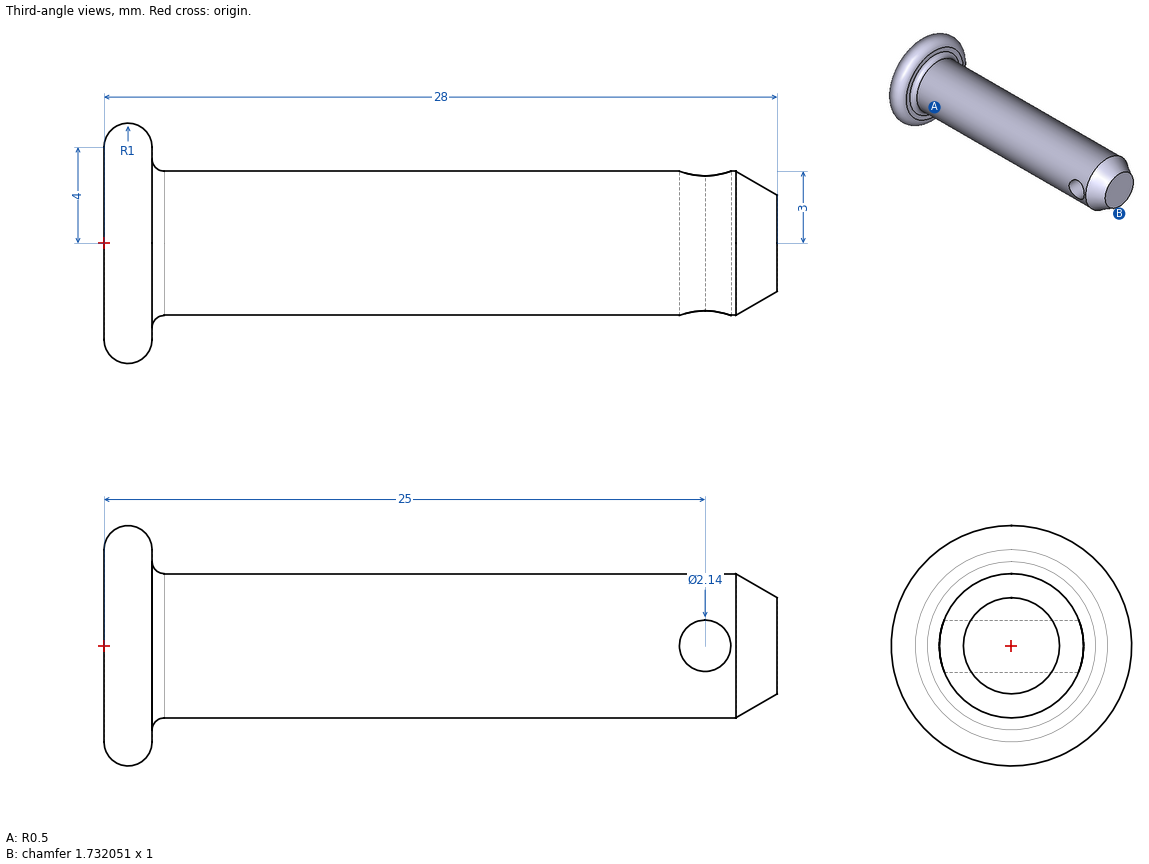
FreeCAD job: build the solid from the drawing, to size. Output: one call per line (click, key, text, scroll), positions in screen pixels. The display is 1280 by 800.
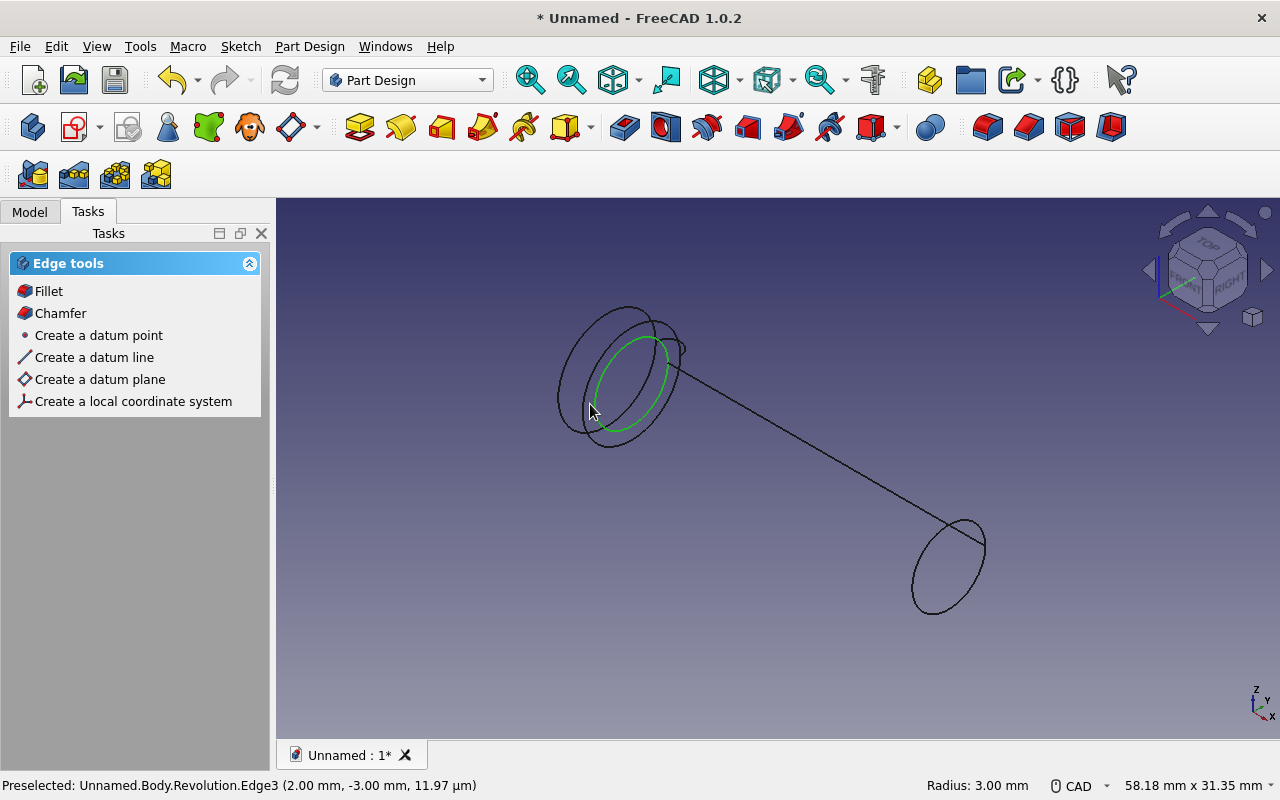
key(v)
key(1)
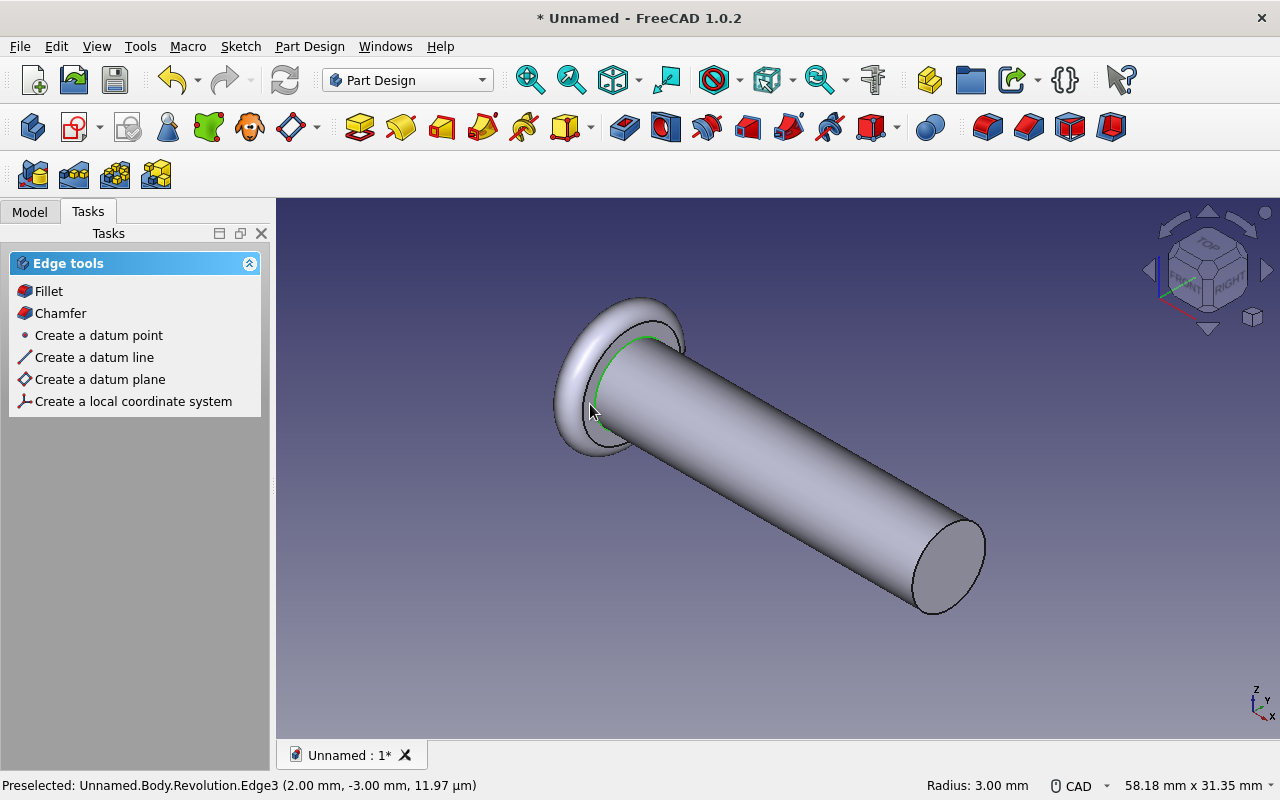
click(988, 128)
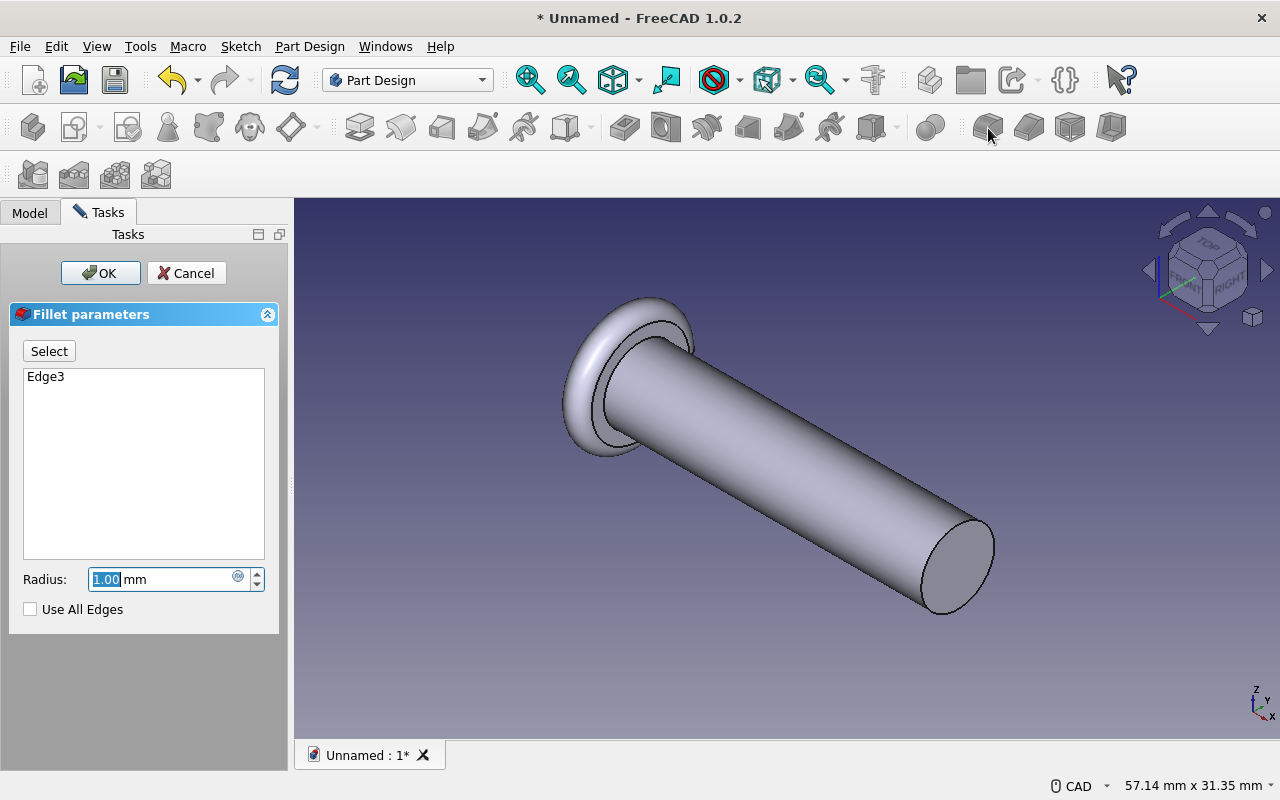
text(0.5)
key(Tab)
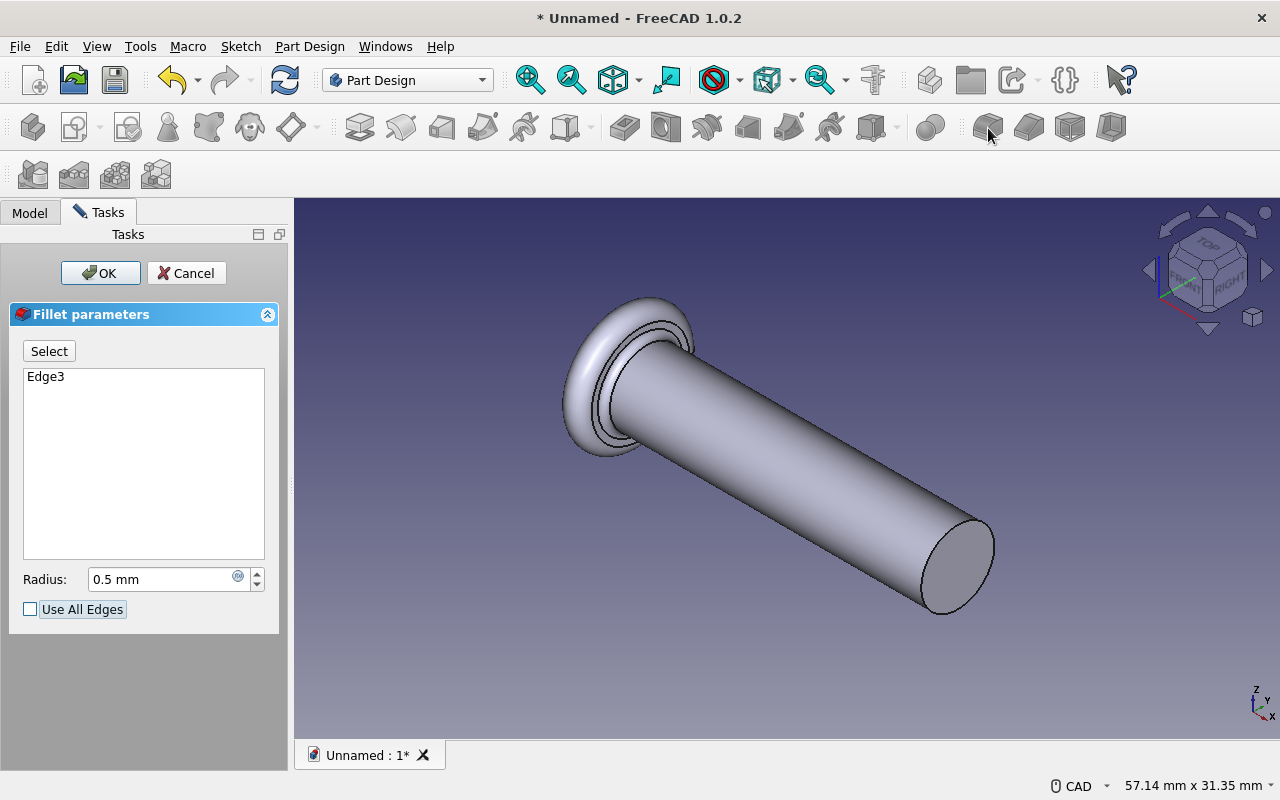
click(101, 273)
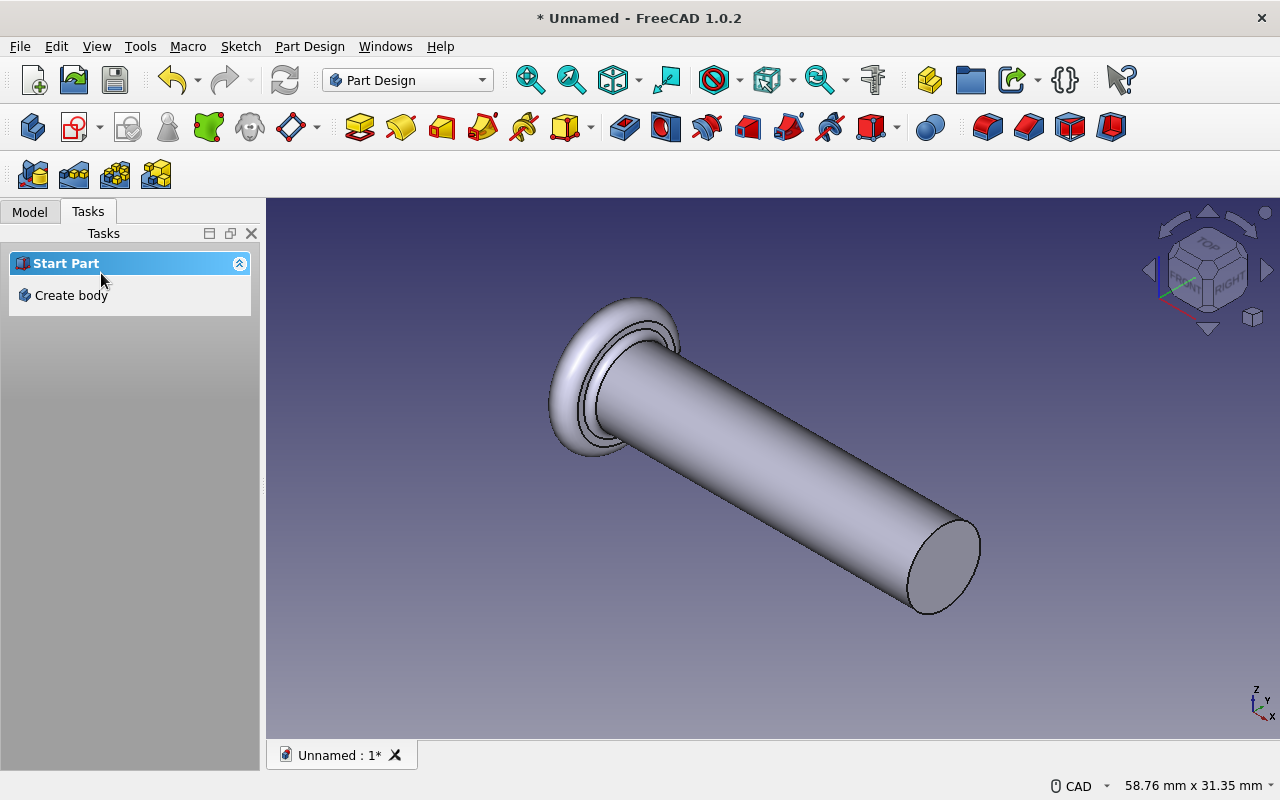
click(907, 587)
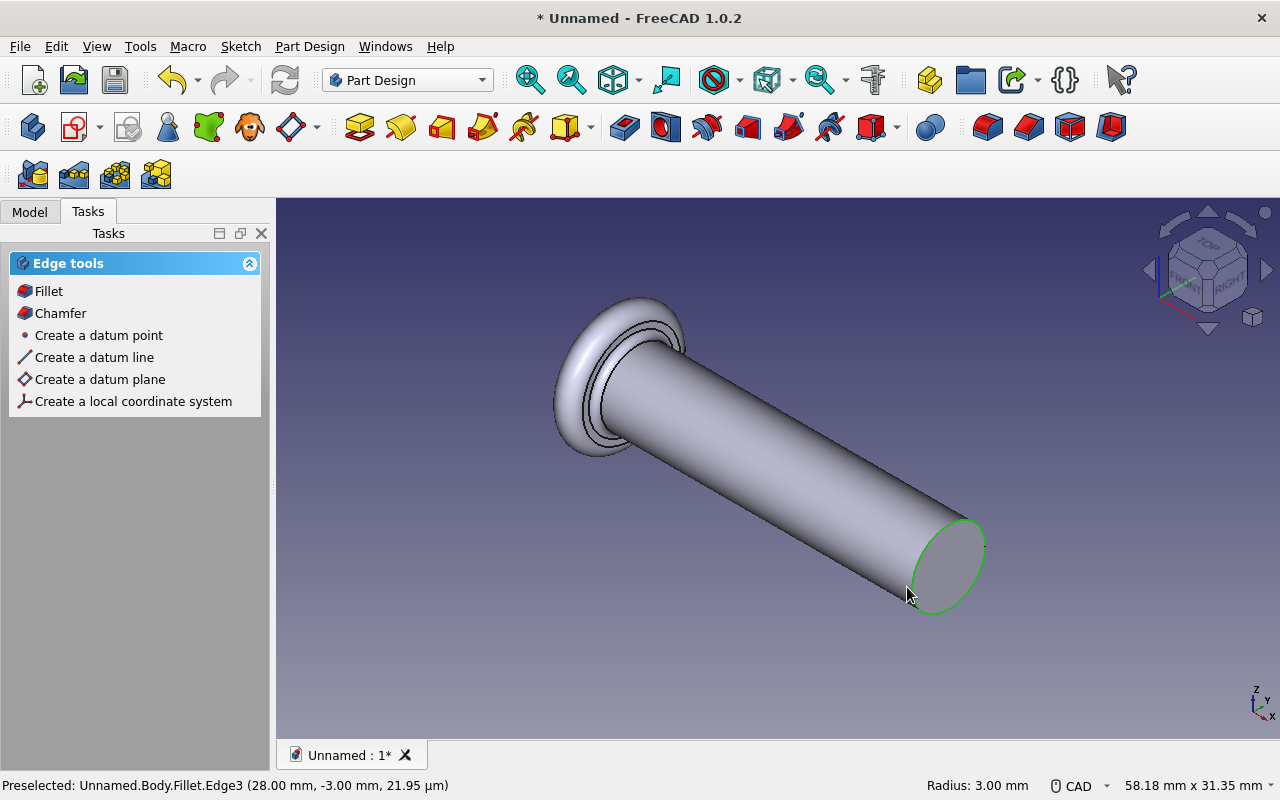
click(1029, 128)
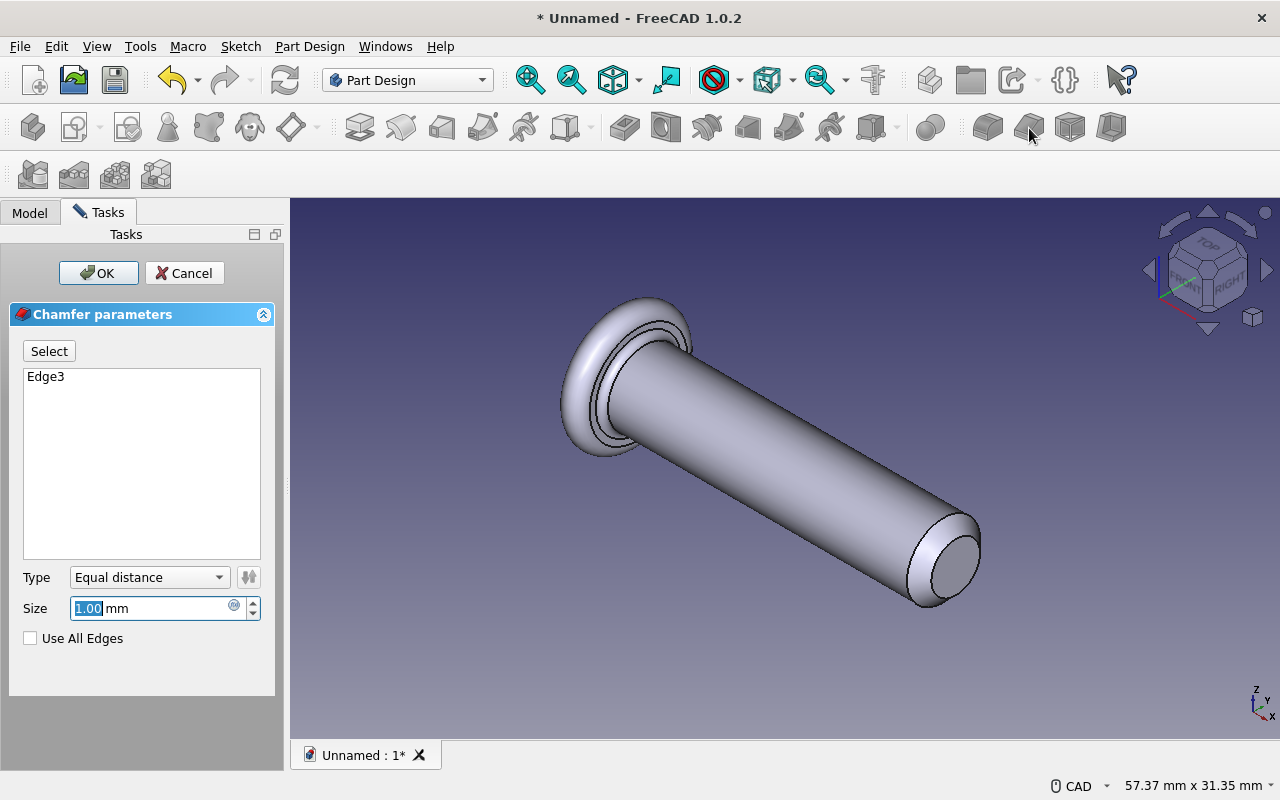
text(1.732051)
key(Tab)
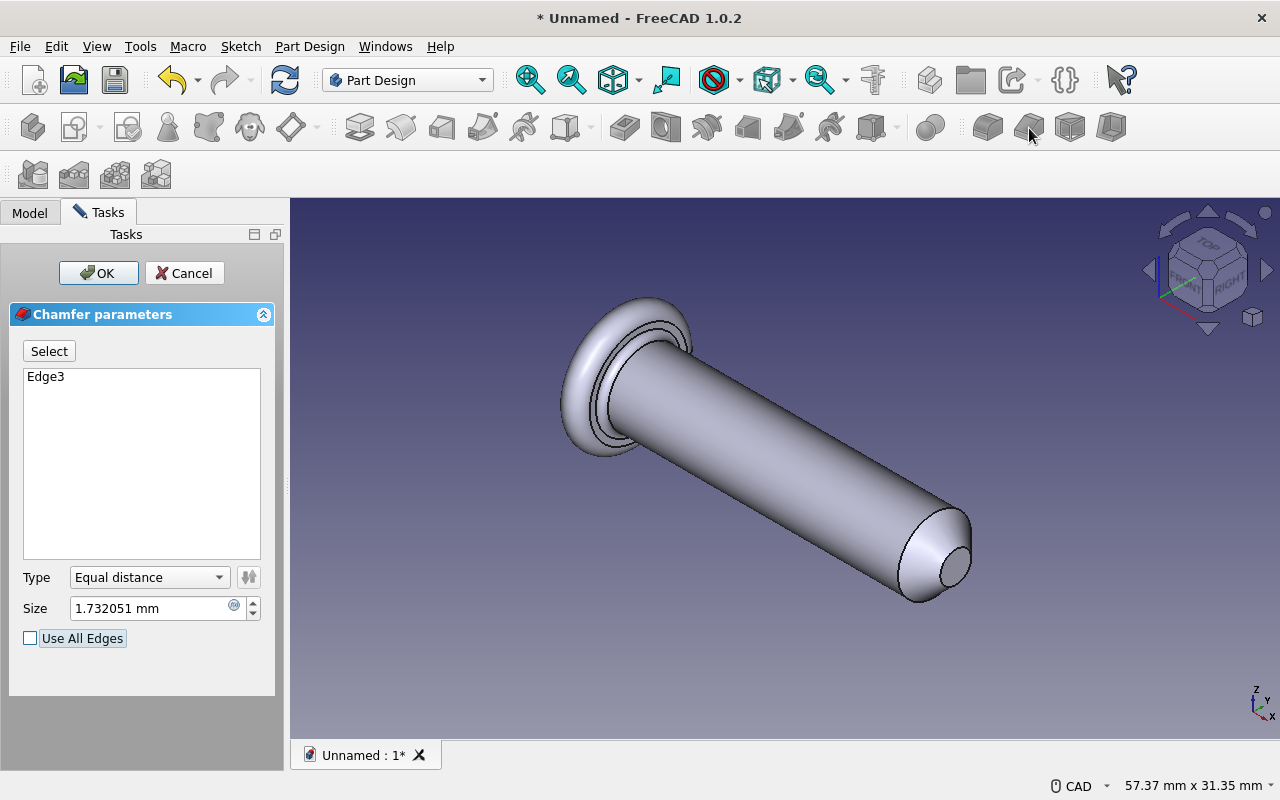
click(150, 578)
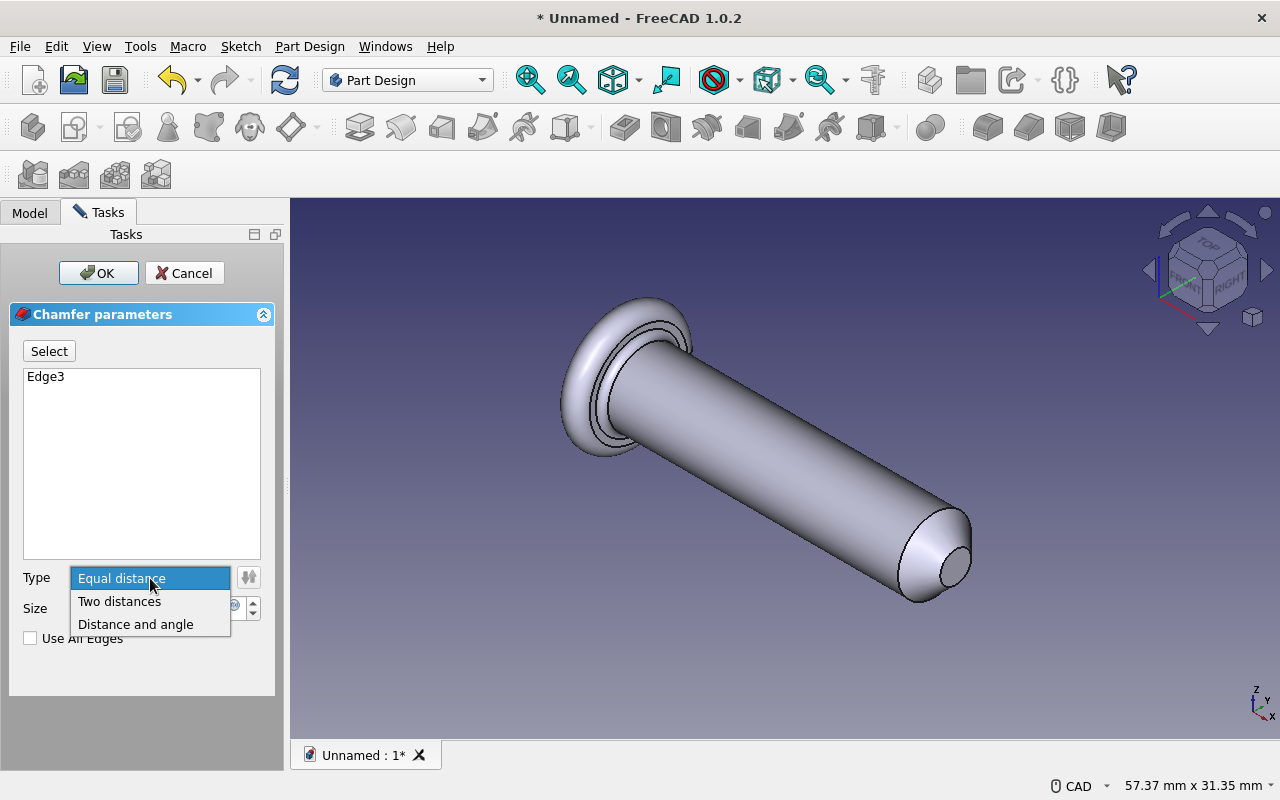
click(148, 602)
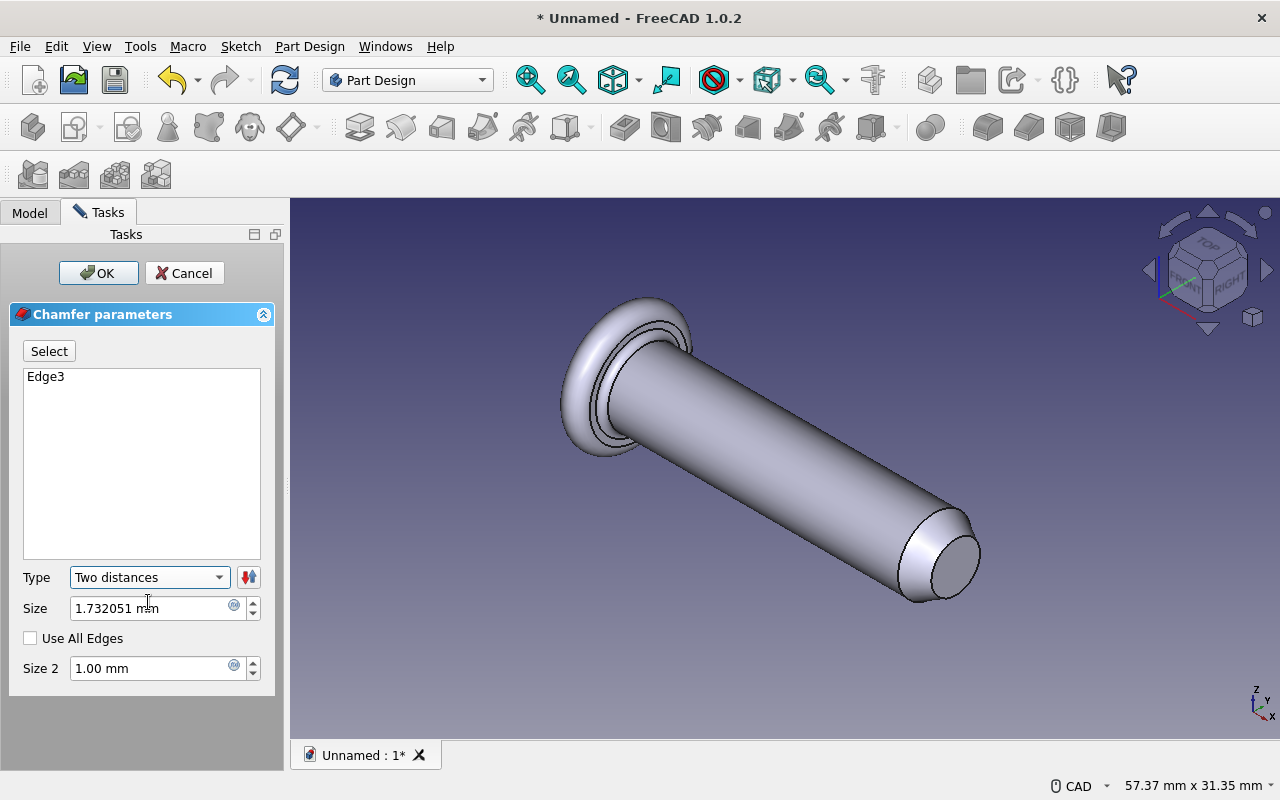
triple_click(158, 668)